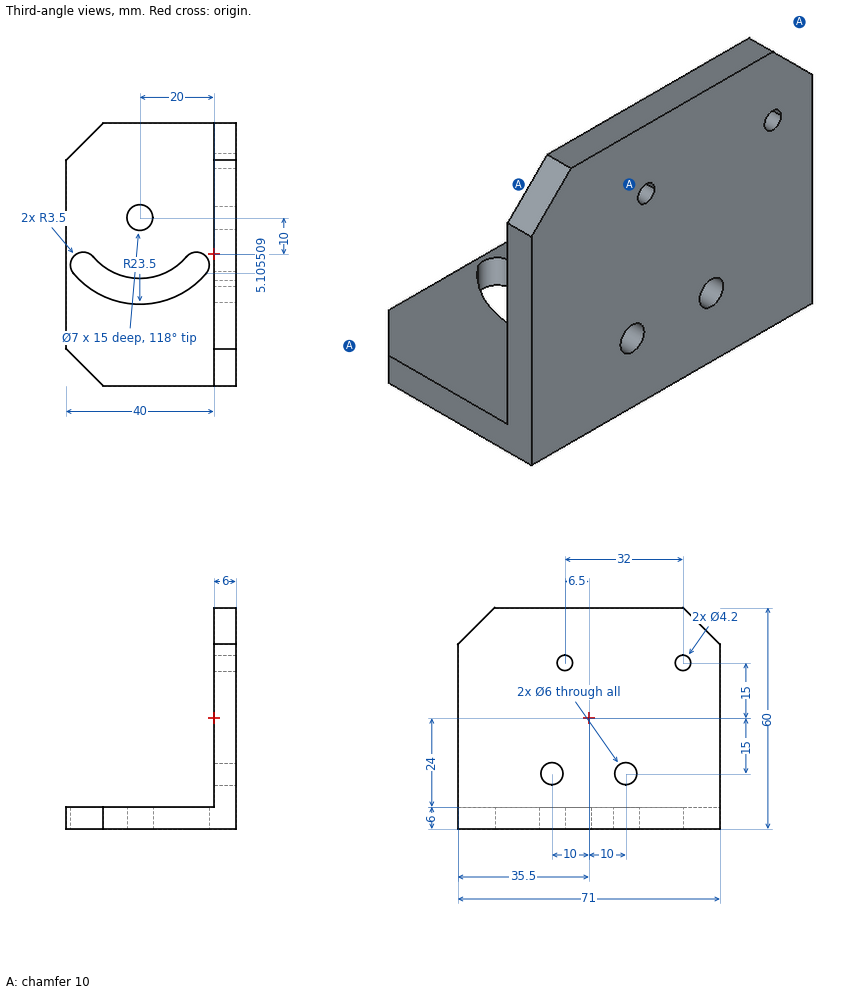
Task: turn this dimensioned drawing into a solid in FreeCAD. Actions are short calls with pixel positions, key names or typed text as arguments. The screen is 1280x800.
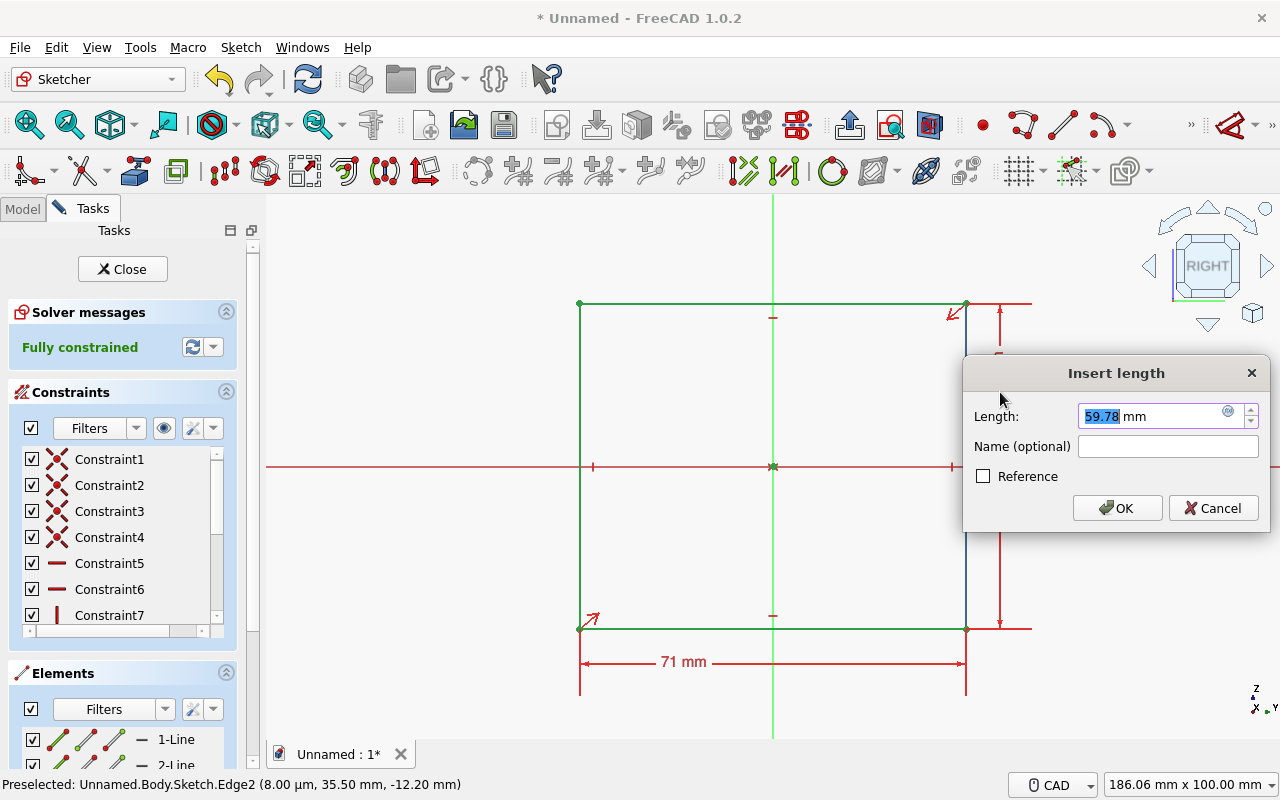
text(60)
key(Return)
key(Escape)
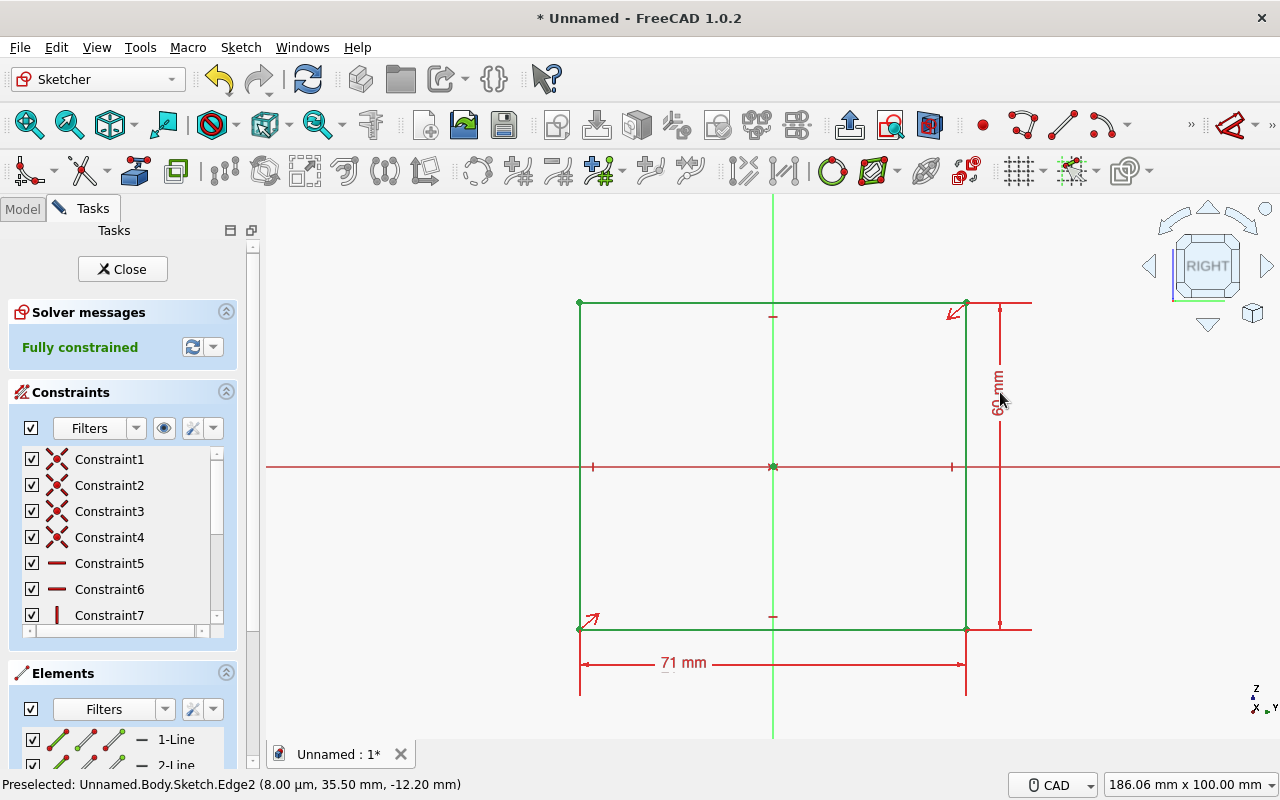
click(123, 269)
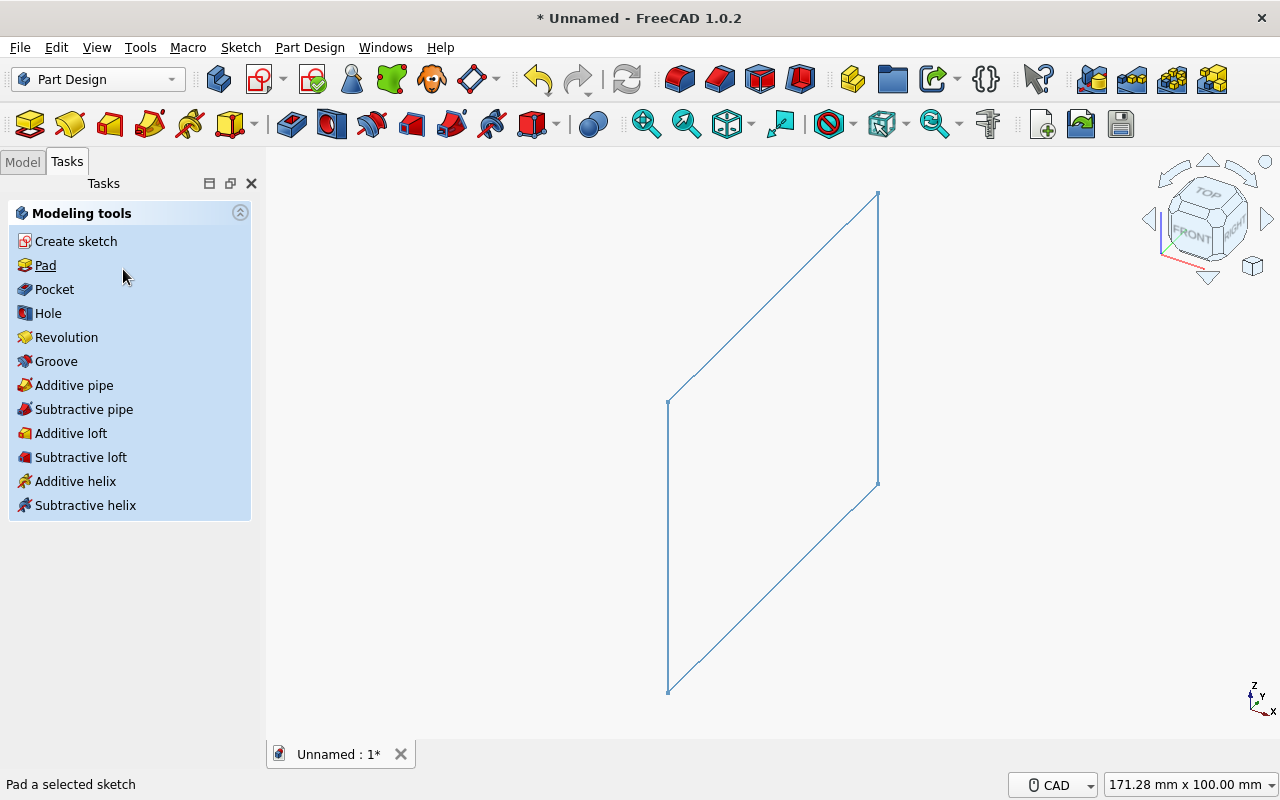
click(30, 124)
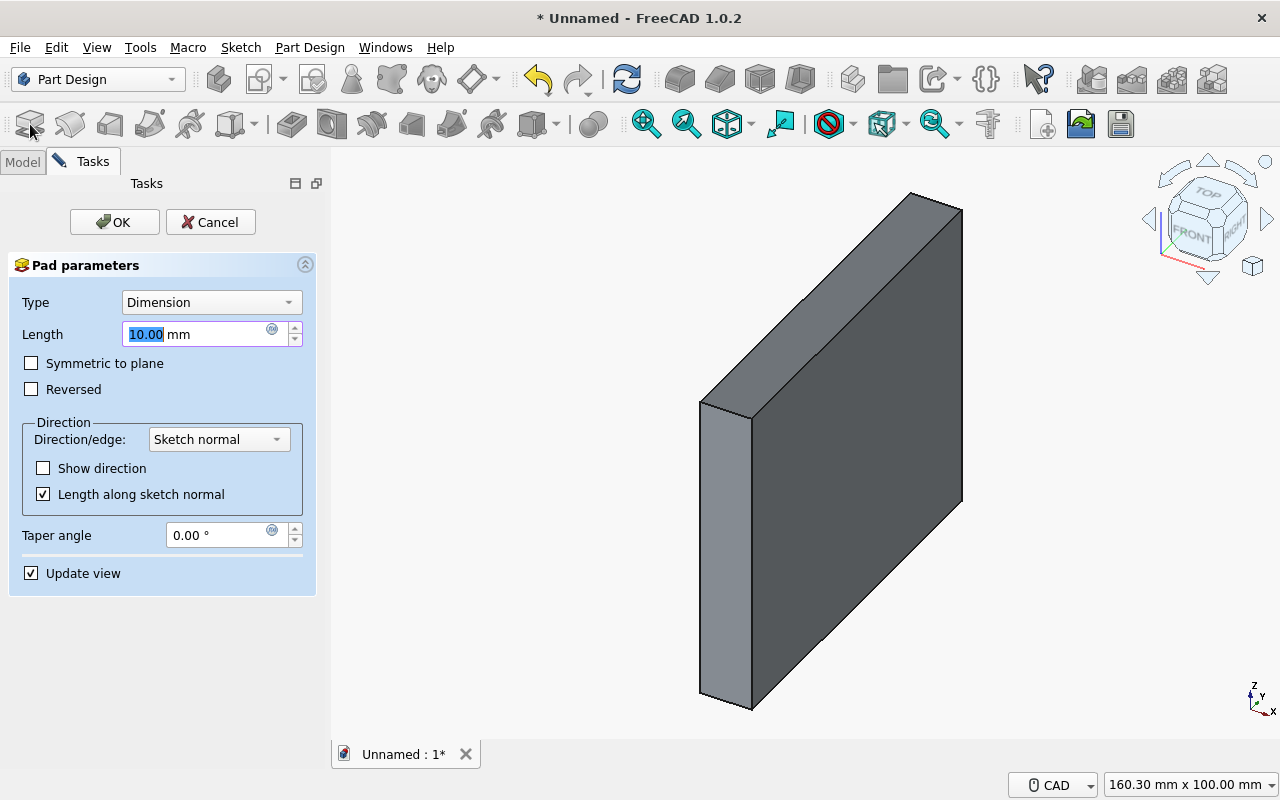
text(6)
key(Tab)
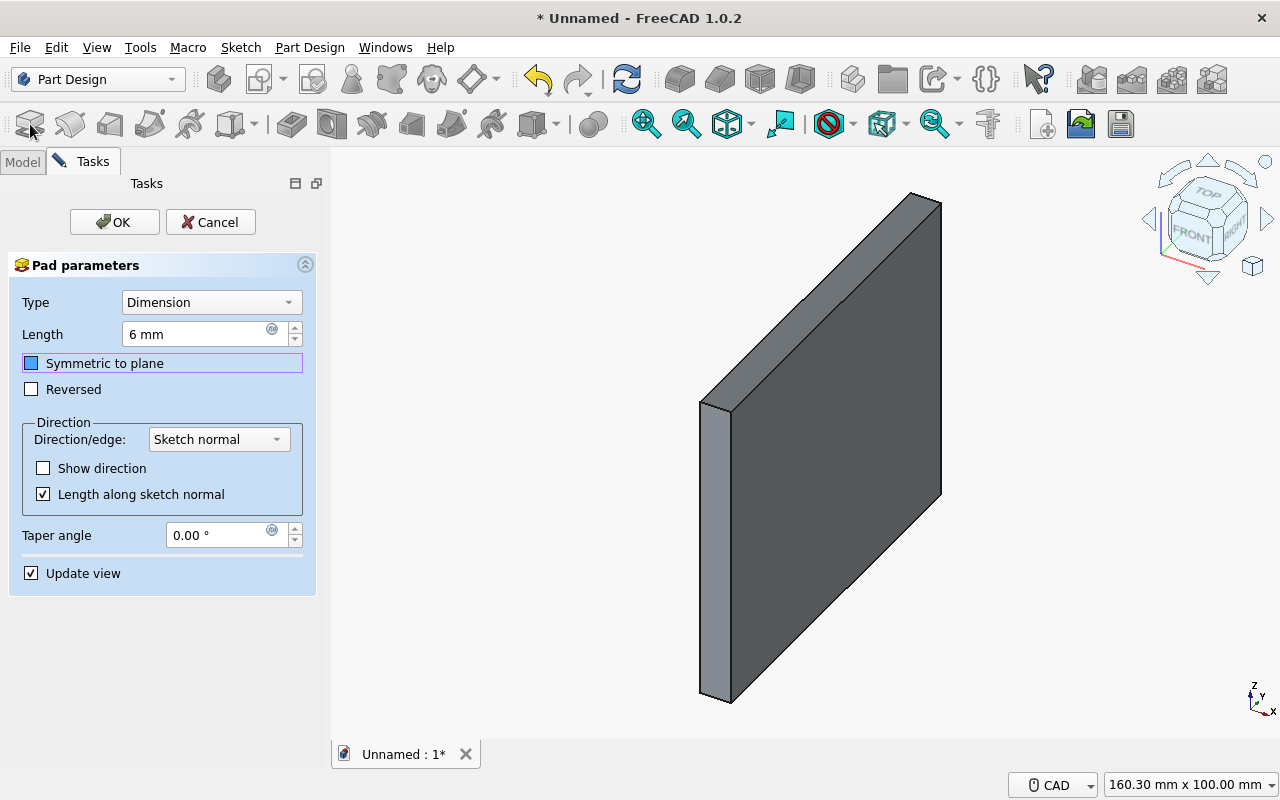
click(115, 222)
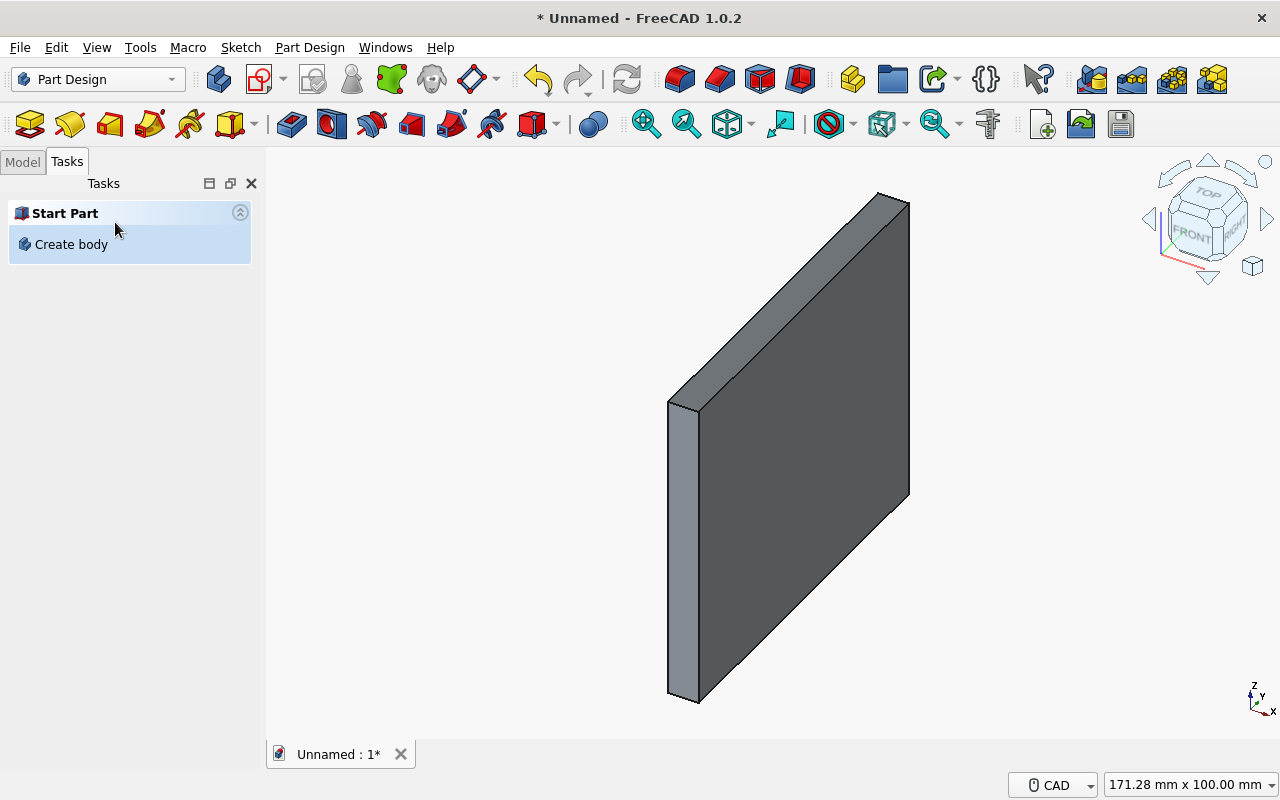
click(804, 452)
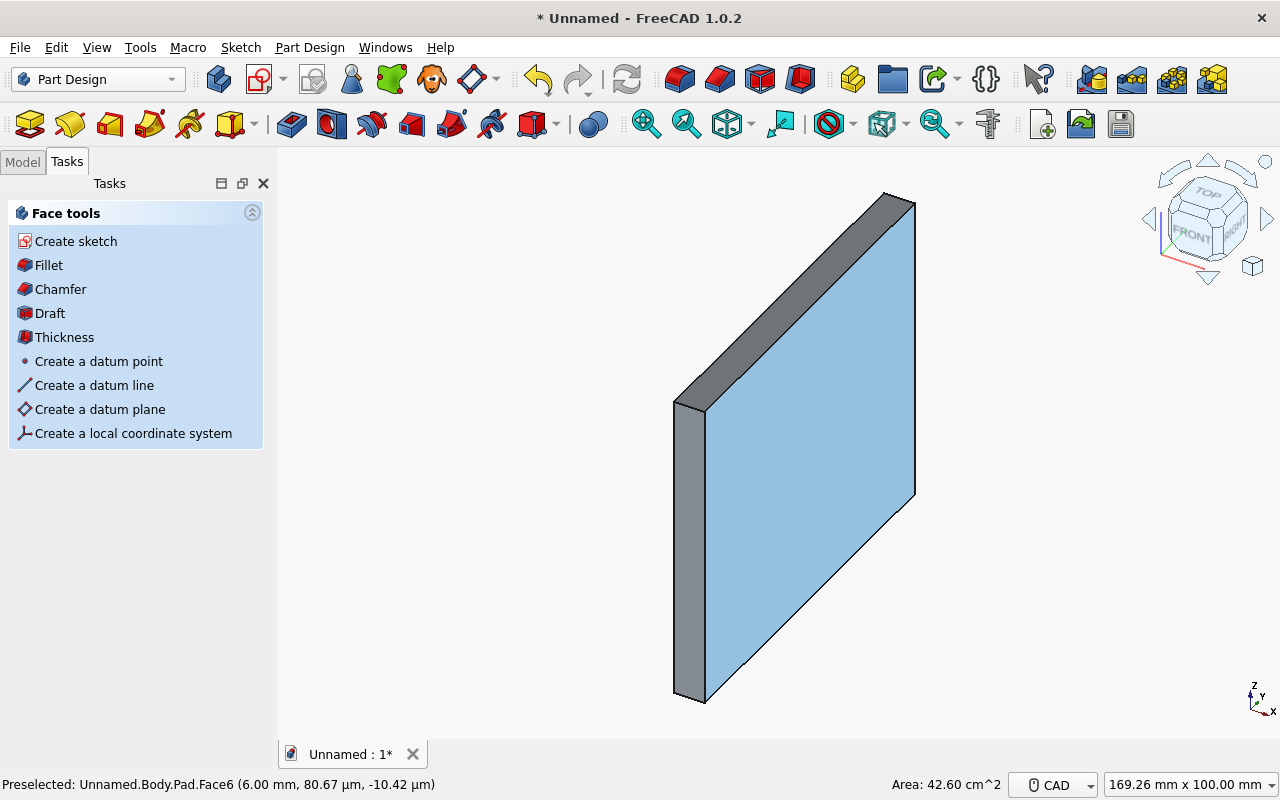
click(260, 80)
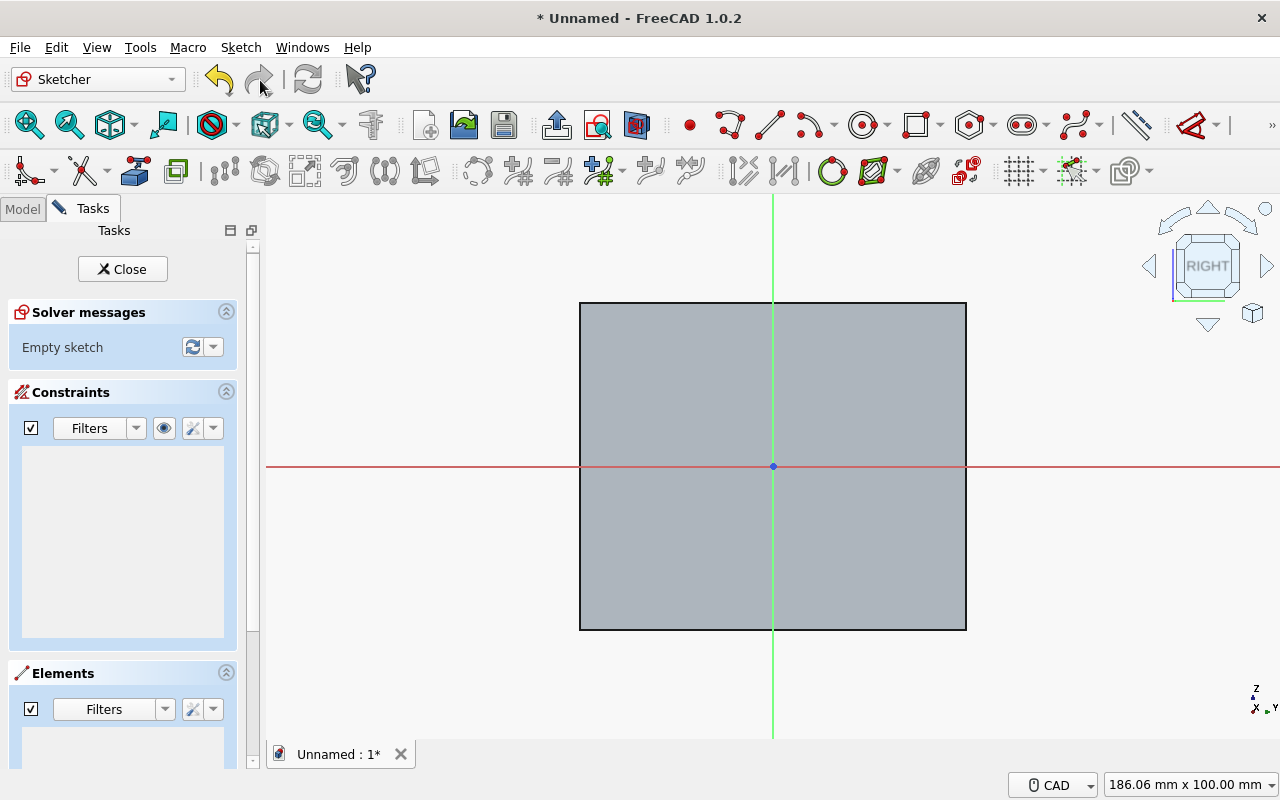
scroll(895, 393, up, 5)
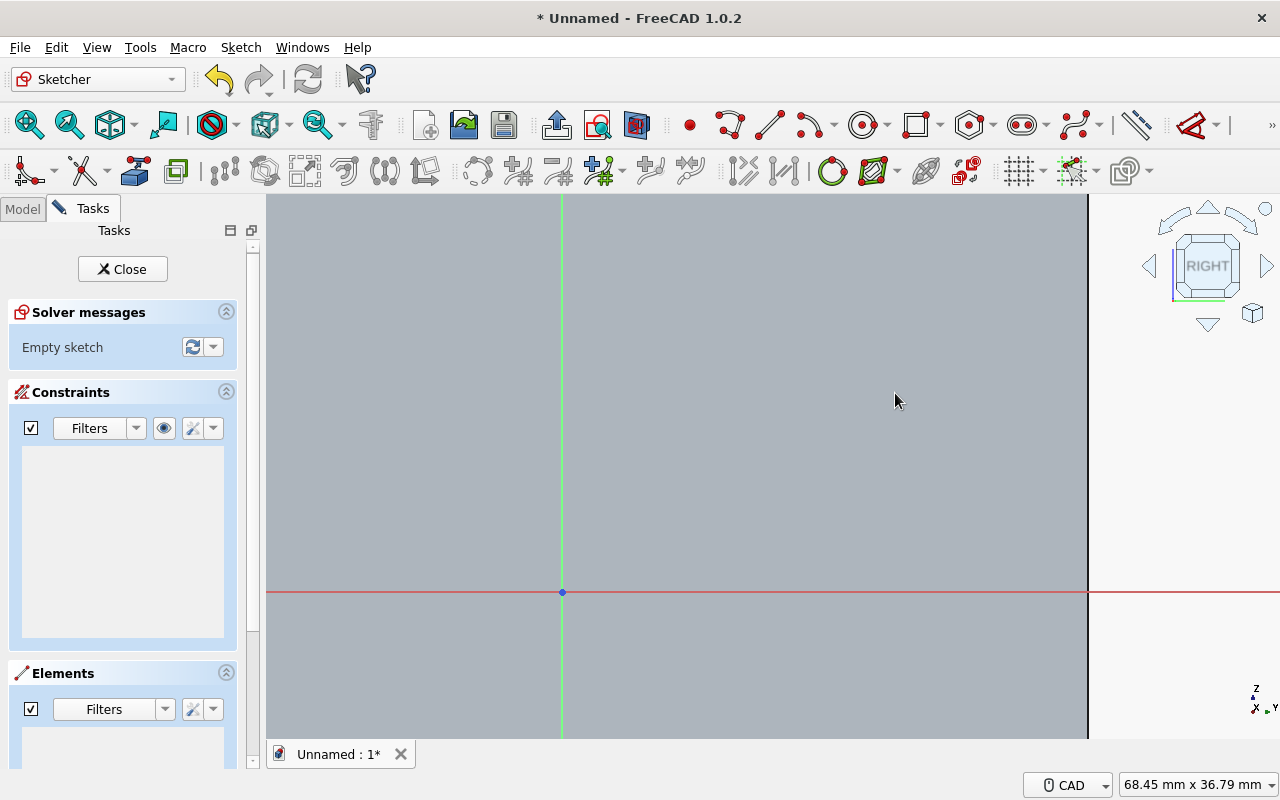
click(864, 126)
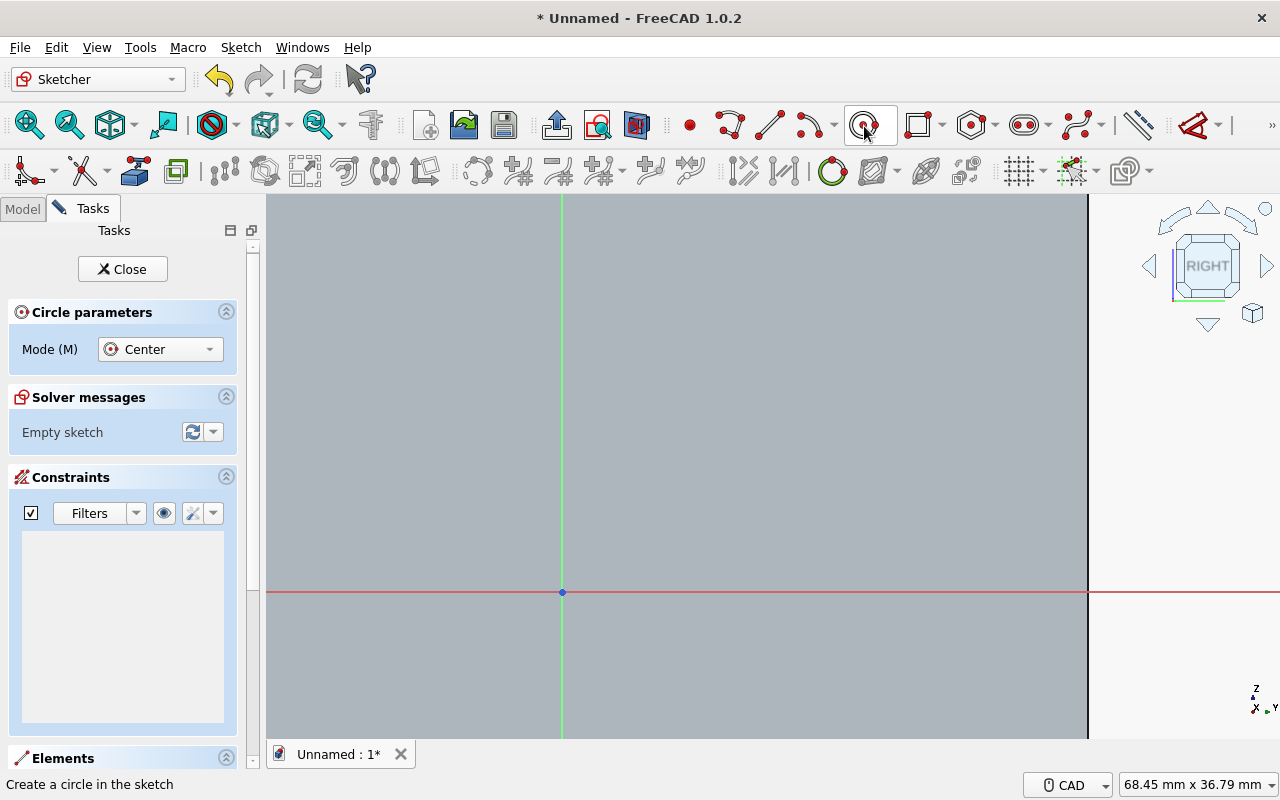
click(940, 370)
click(962, 348)